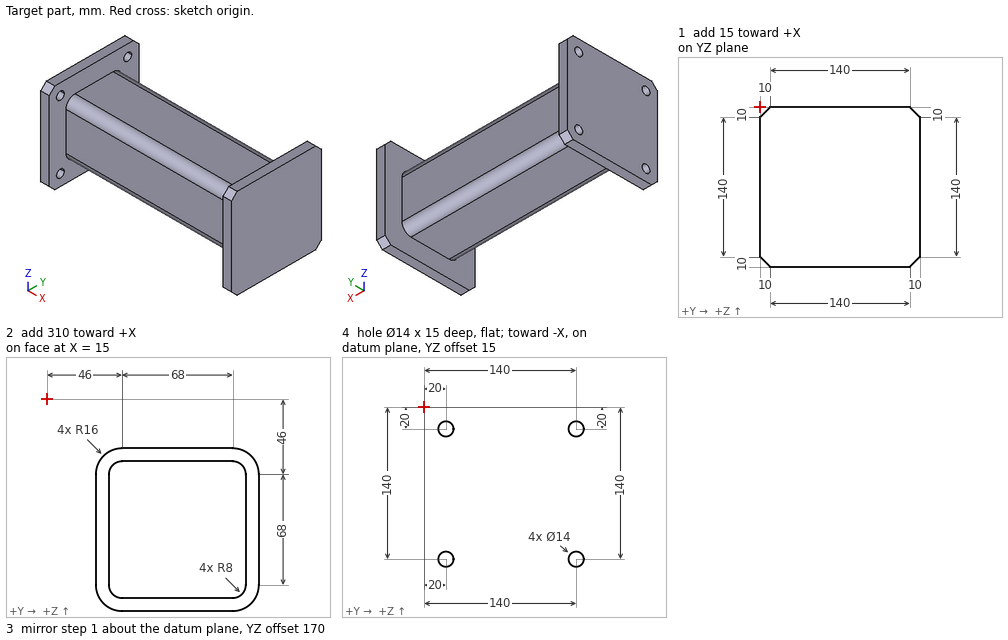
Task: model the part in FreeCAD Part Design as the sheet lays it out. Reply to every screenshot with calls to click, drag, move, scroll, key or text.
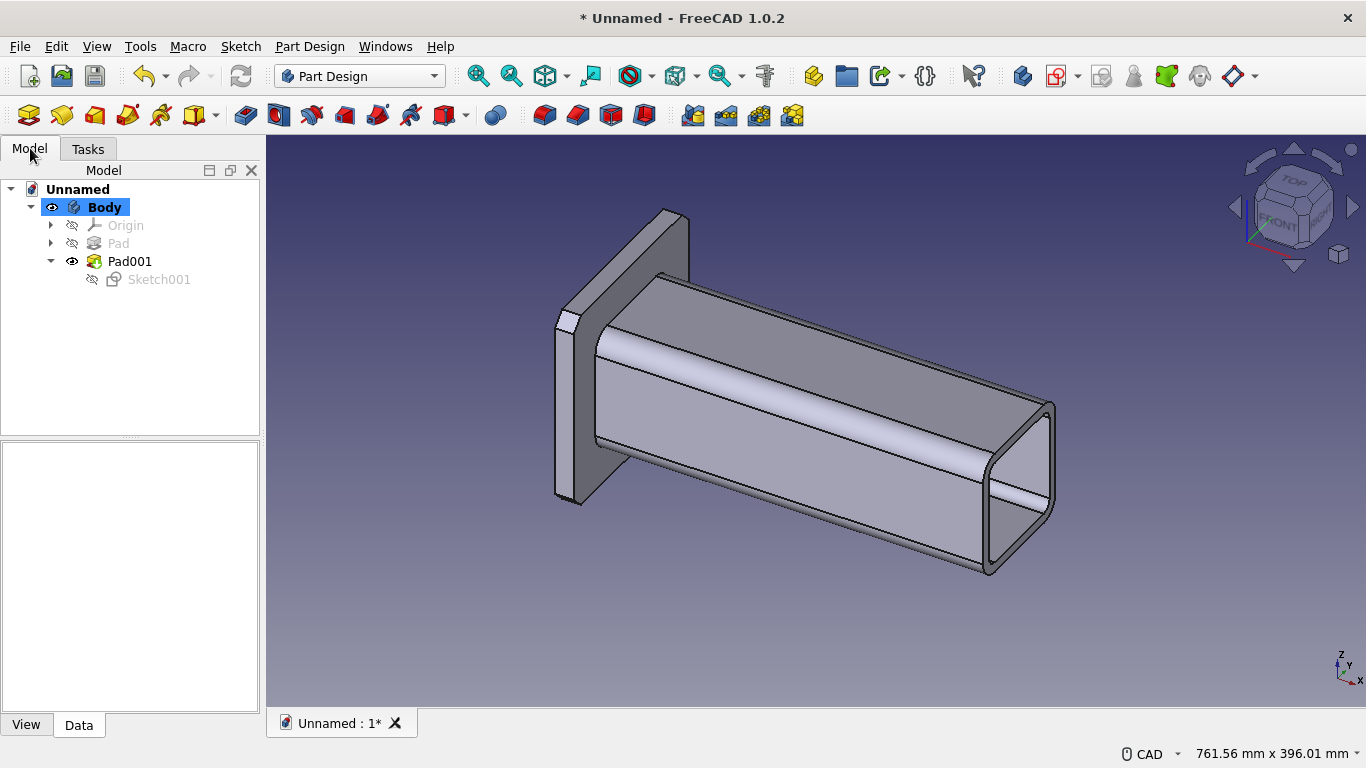
click(51, 225)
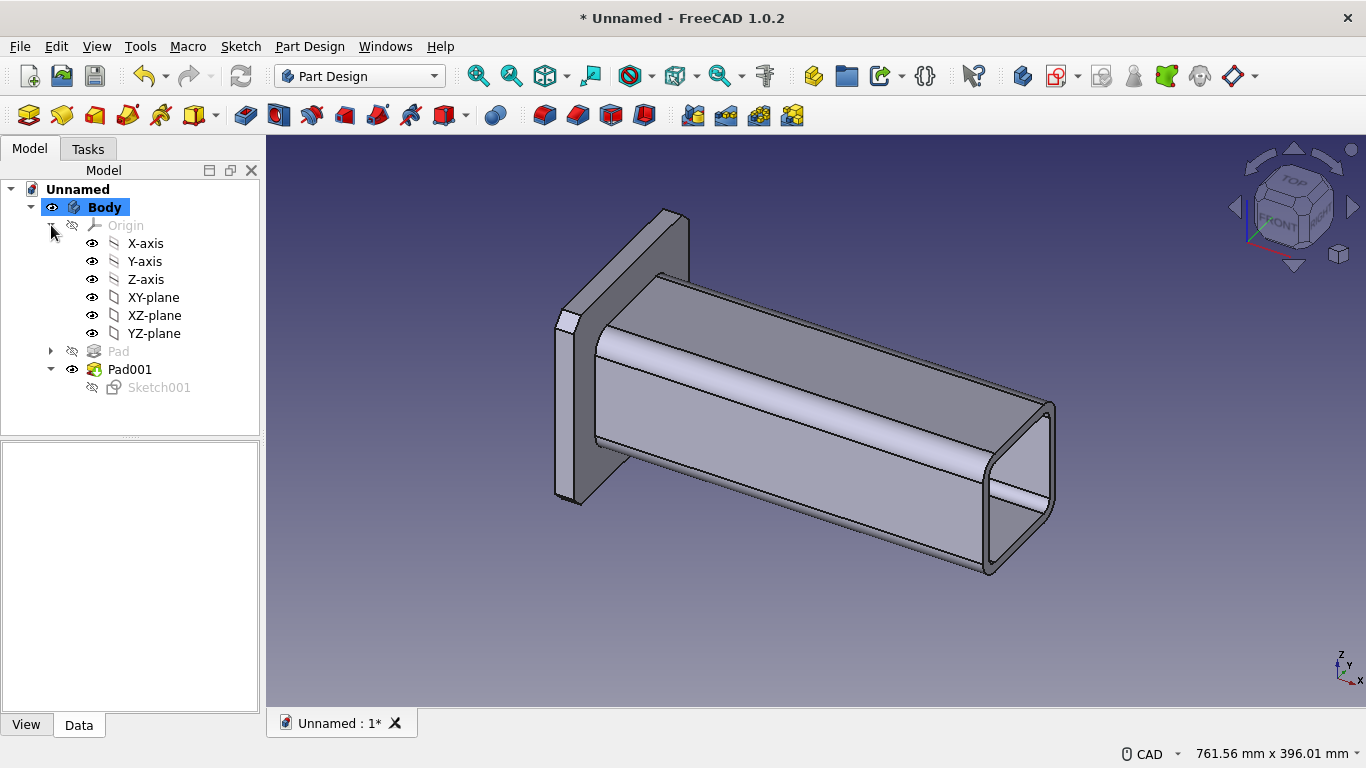
click(137, 333)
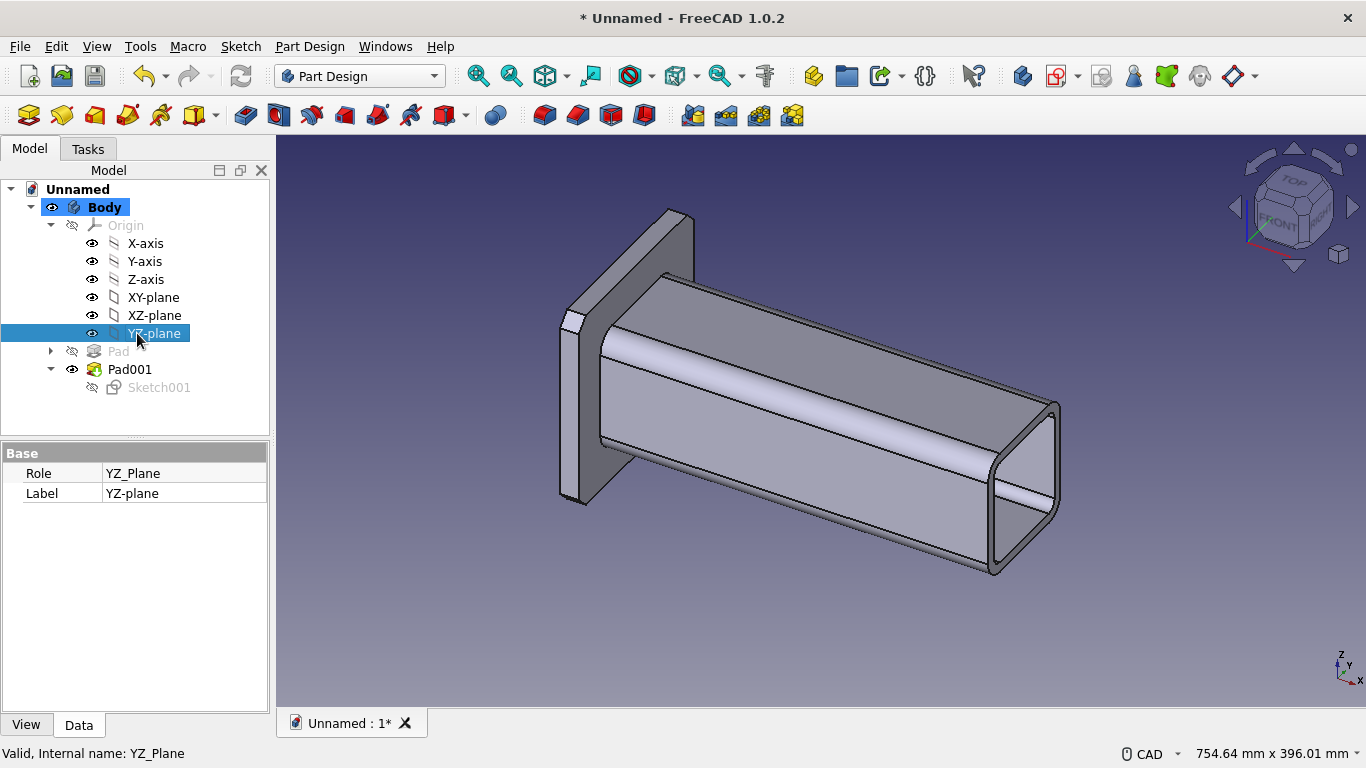
click(1232, 76)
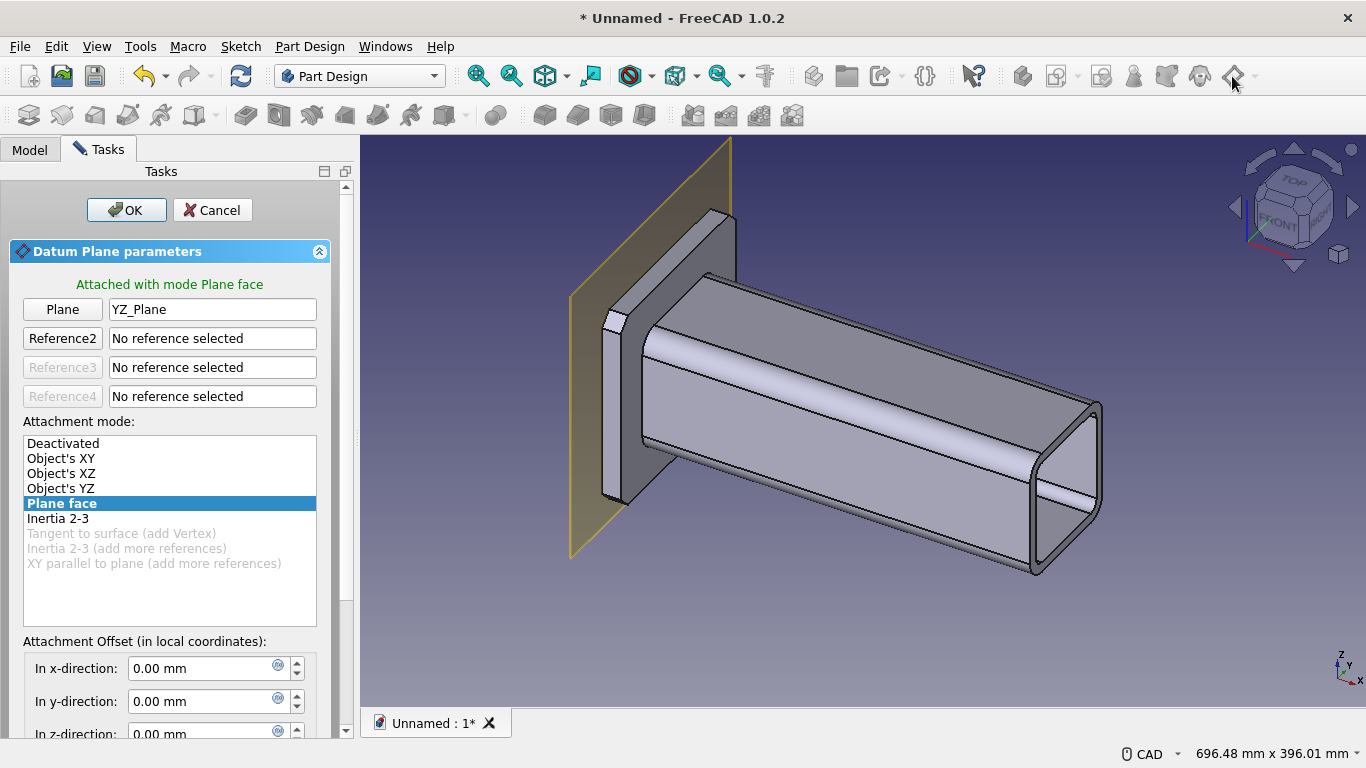
scroll(346, 460, down, 2)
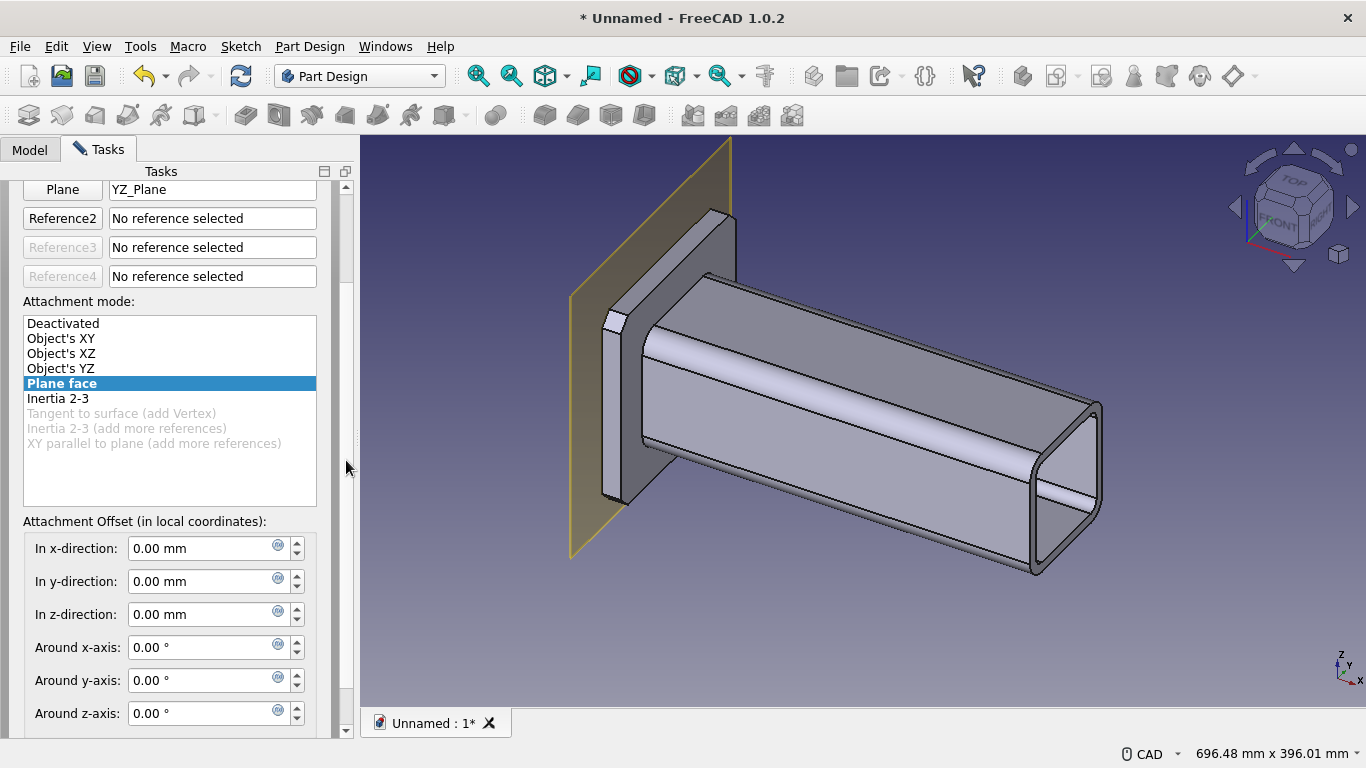
triple_click(210, 614)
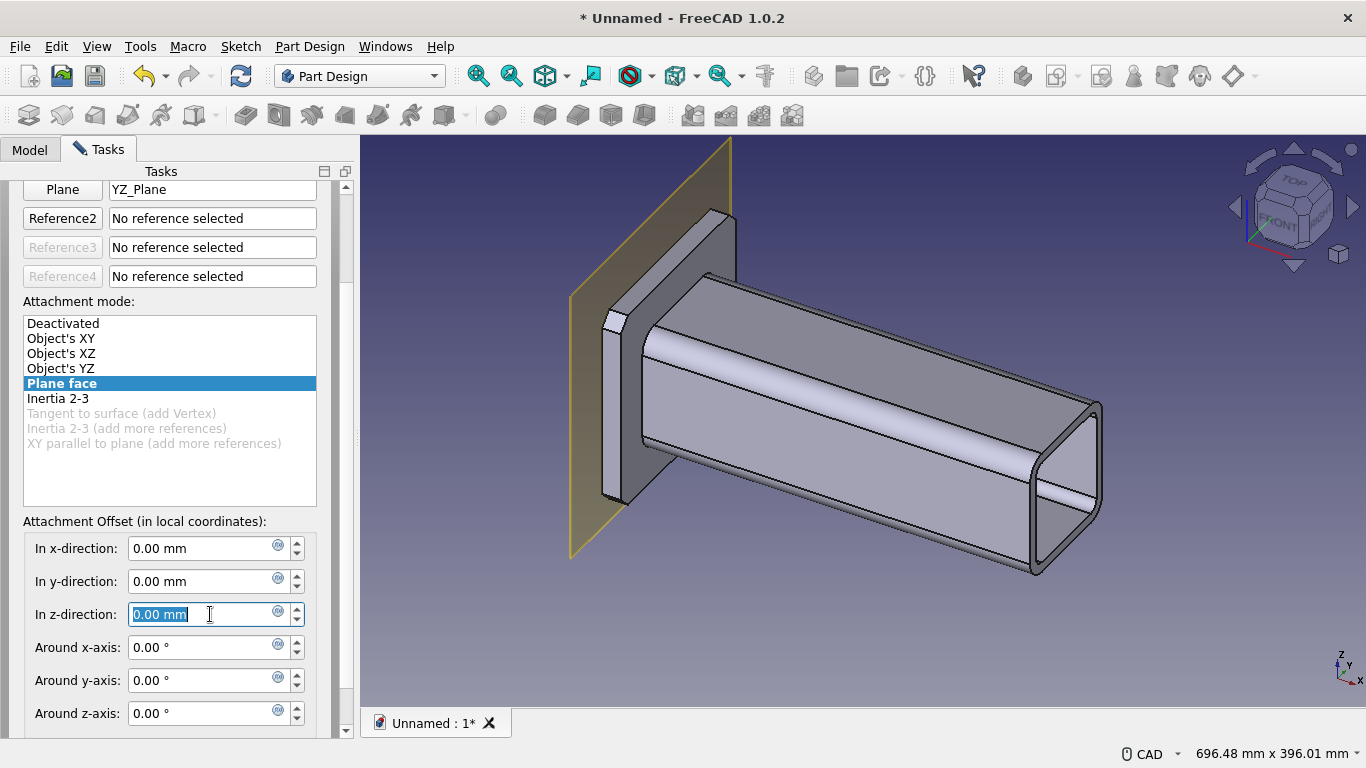
text(170)
key(Tab)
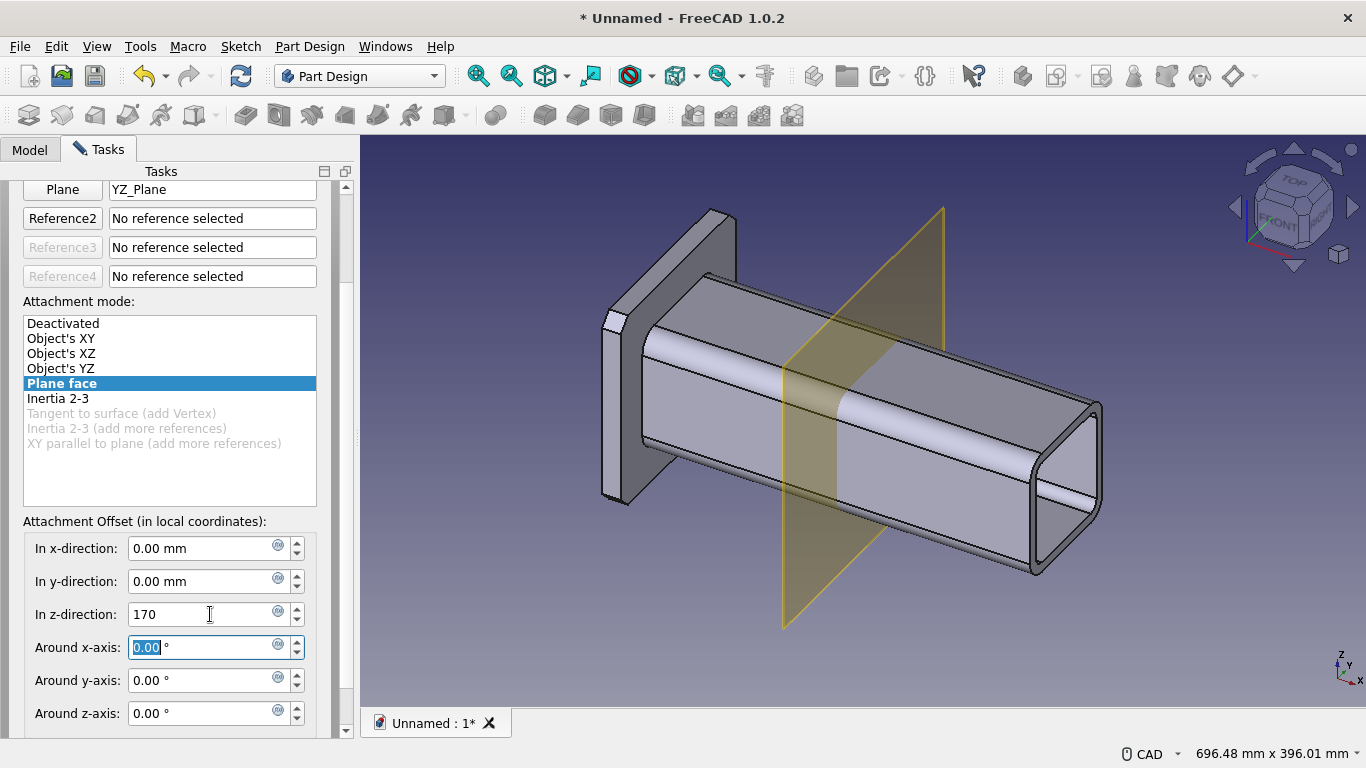
scroll(346, 460, up, 3)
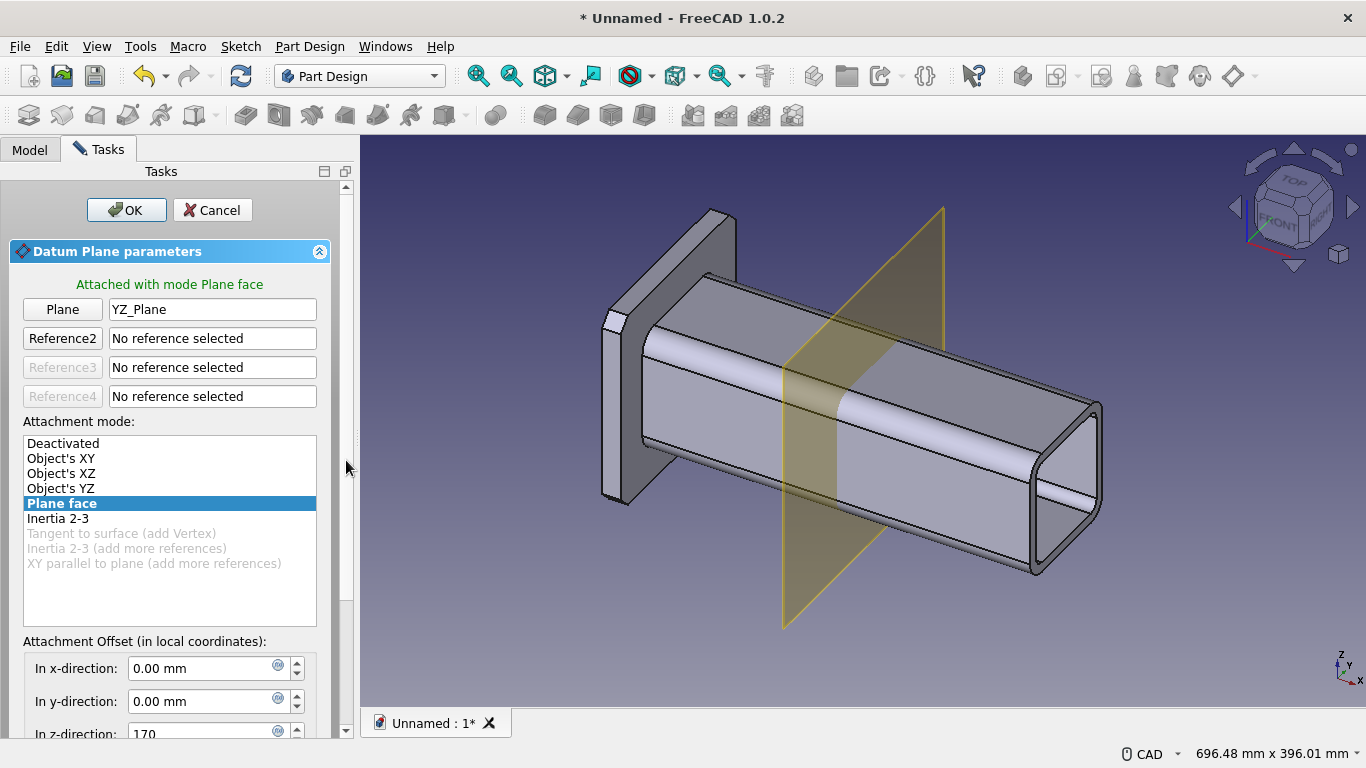
click(127, 210)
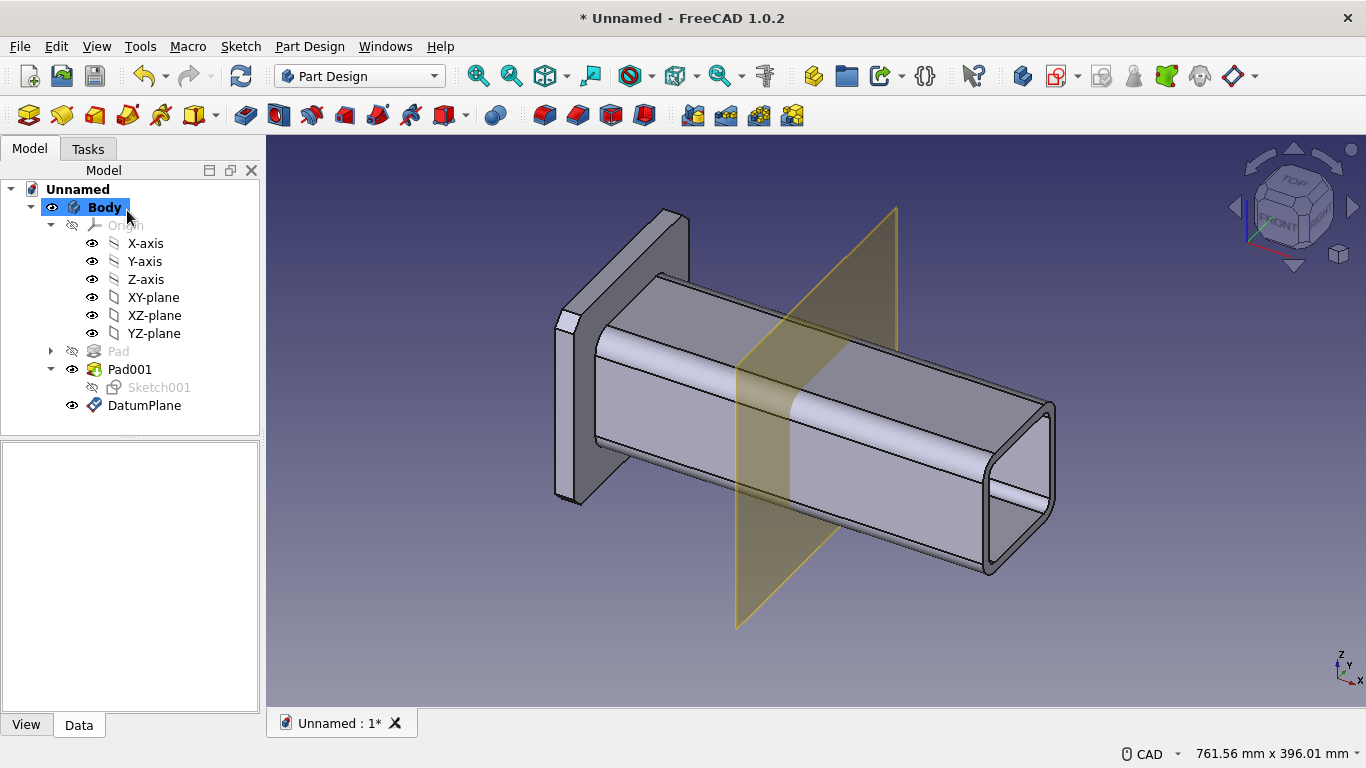
click(117, 351)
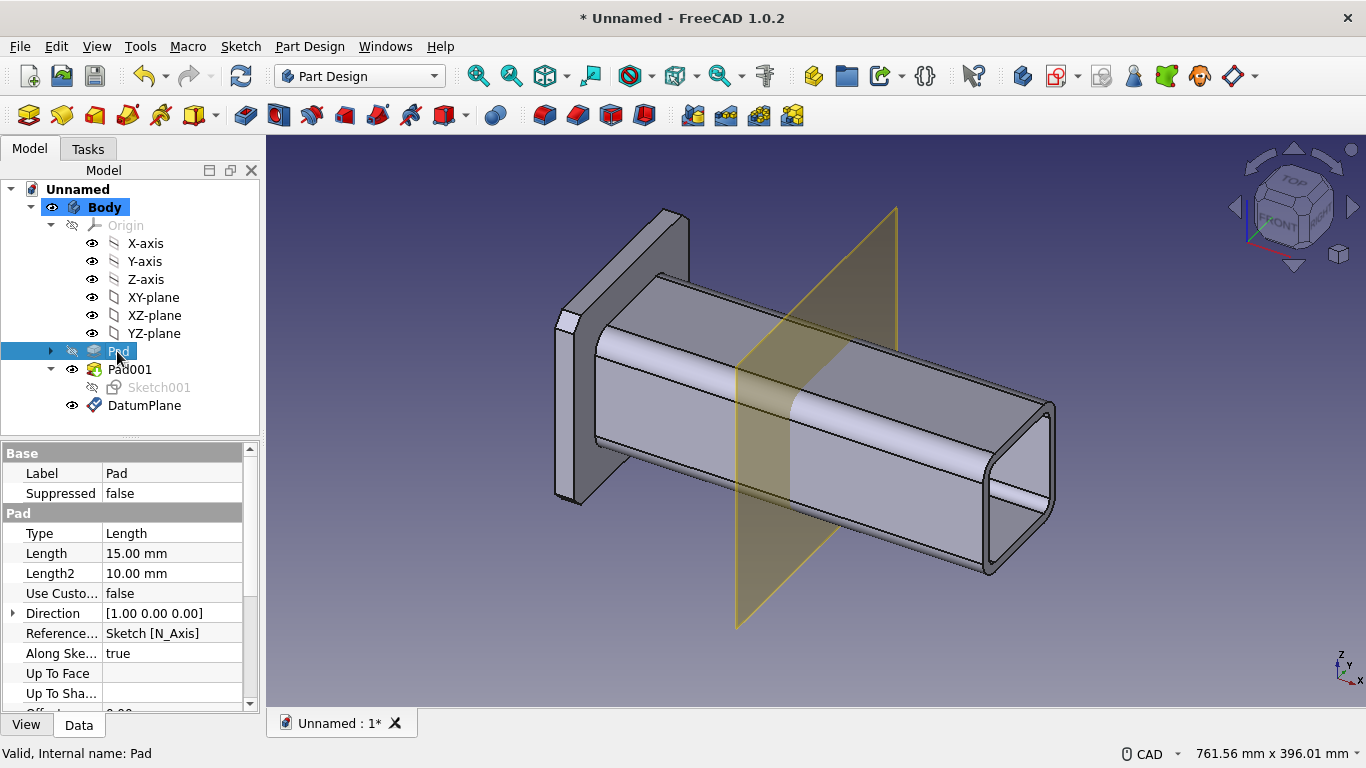
click(693, 116)